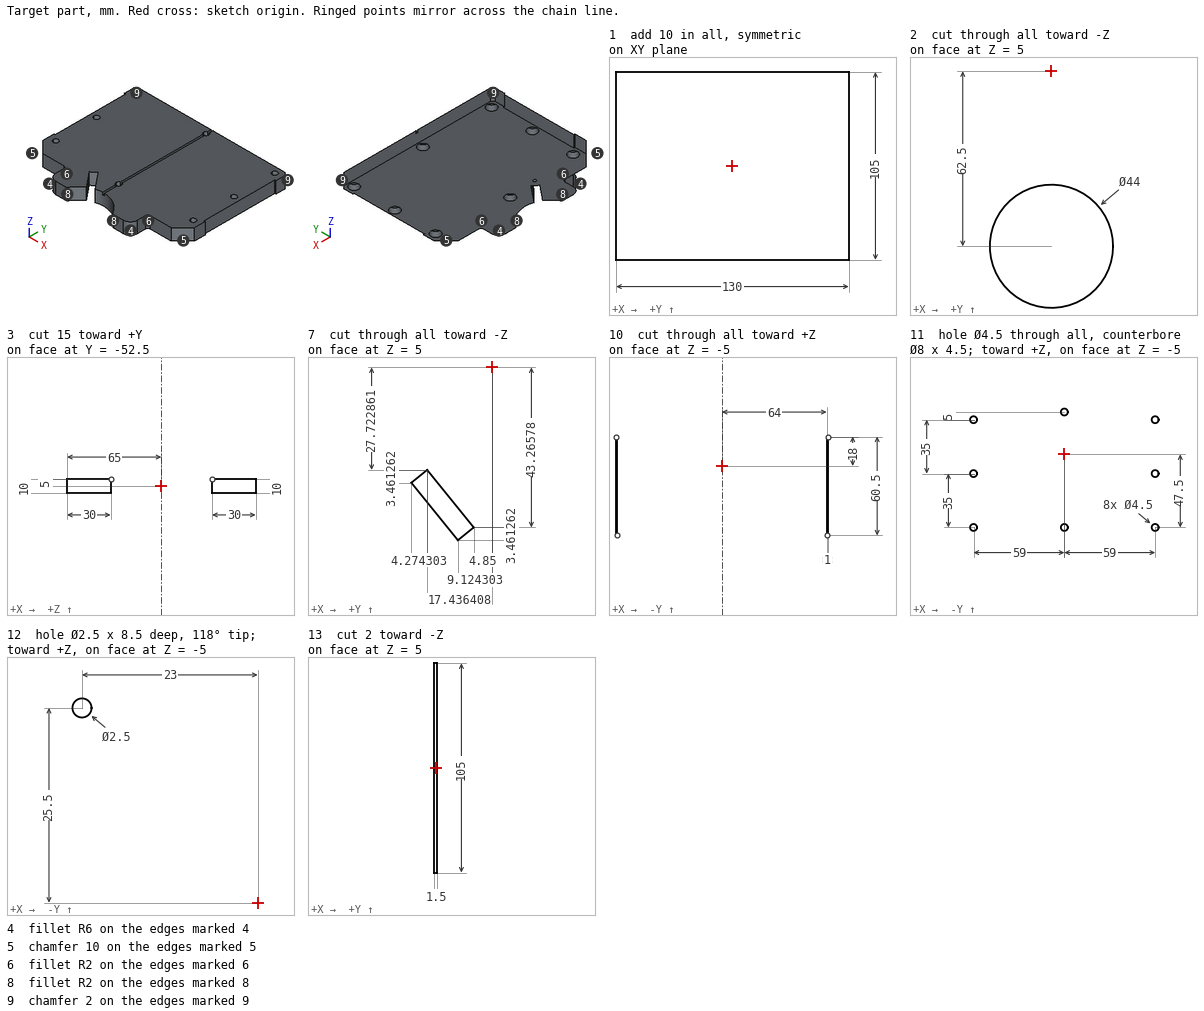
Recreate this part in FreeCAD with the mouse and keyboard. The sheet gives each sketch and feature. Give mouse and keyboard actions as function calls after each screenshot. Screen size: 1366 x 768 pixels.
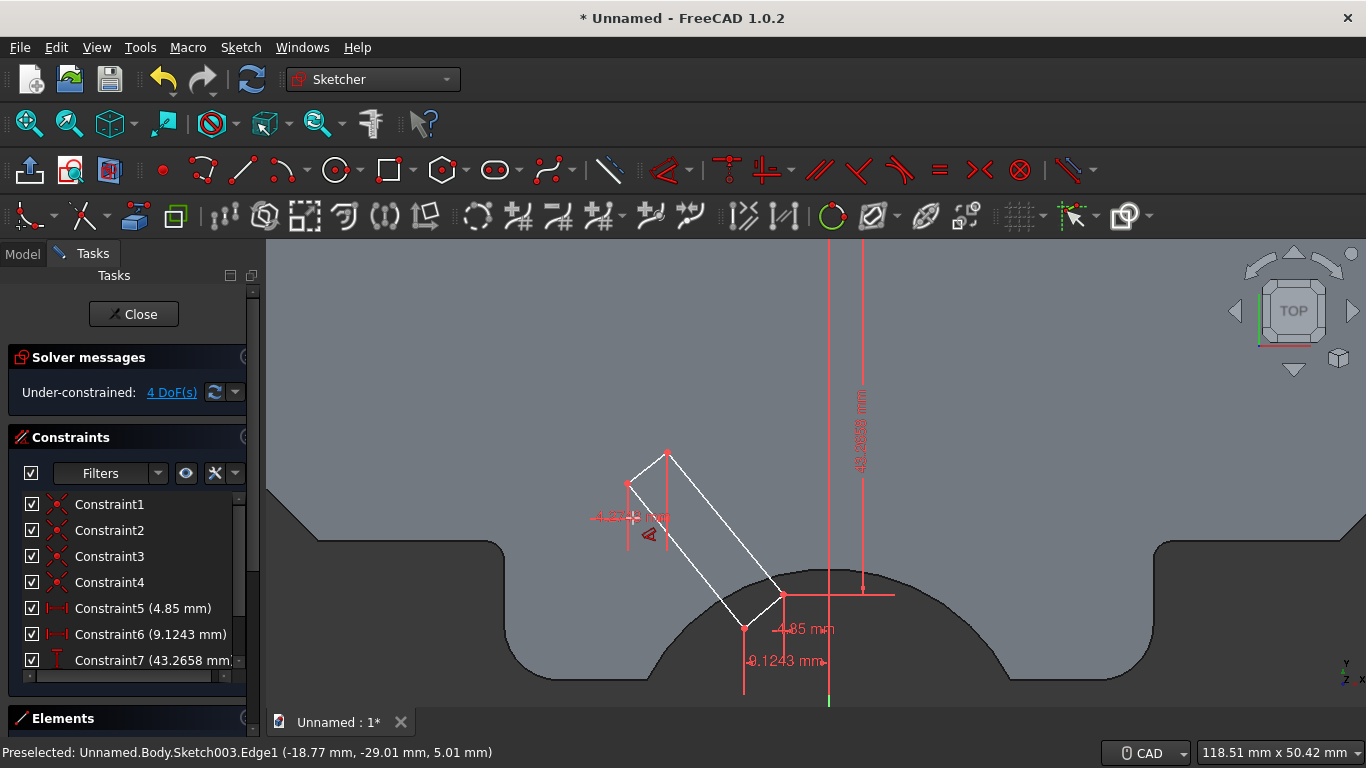
scroll(656, 462, up, 2)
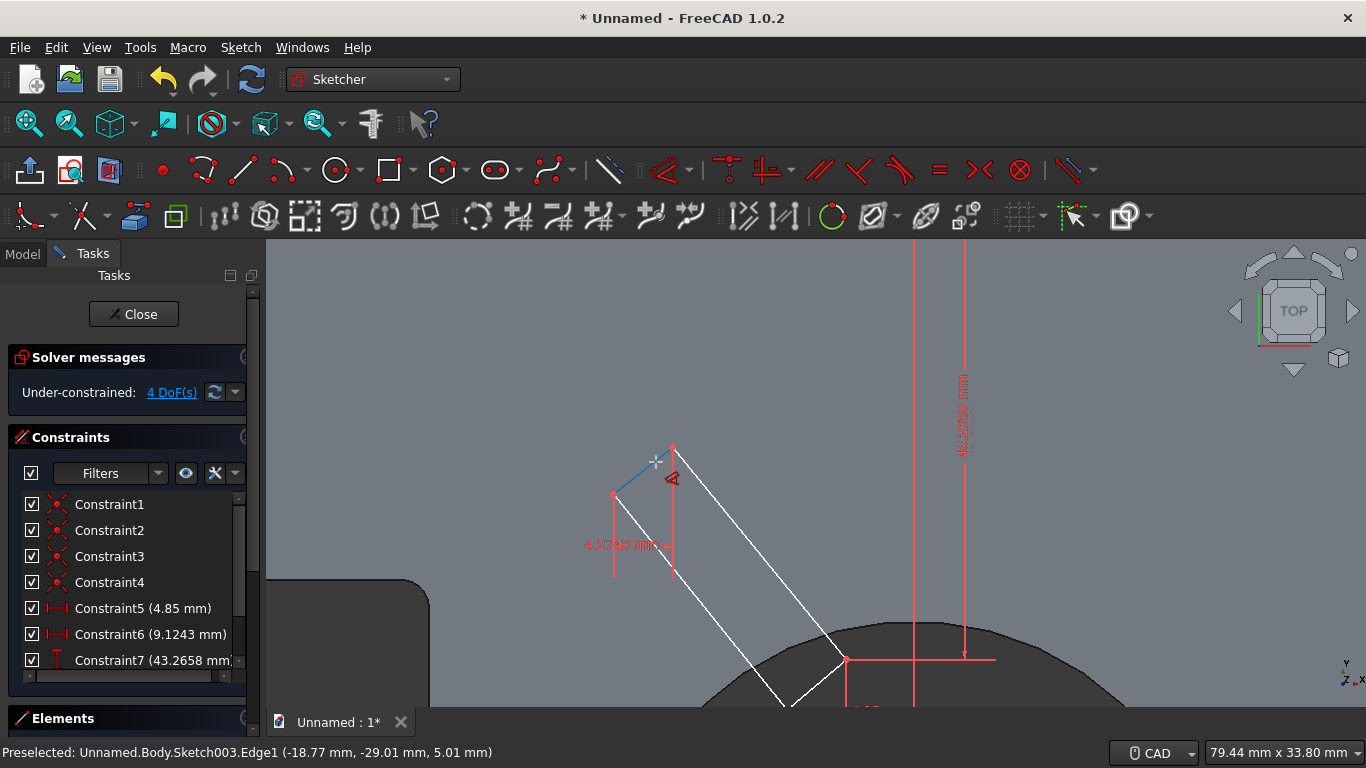
click(655, 461)
click(580, 471)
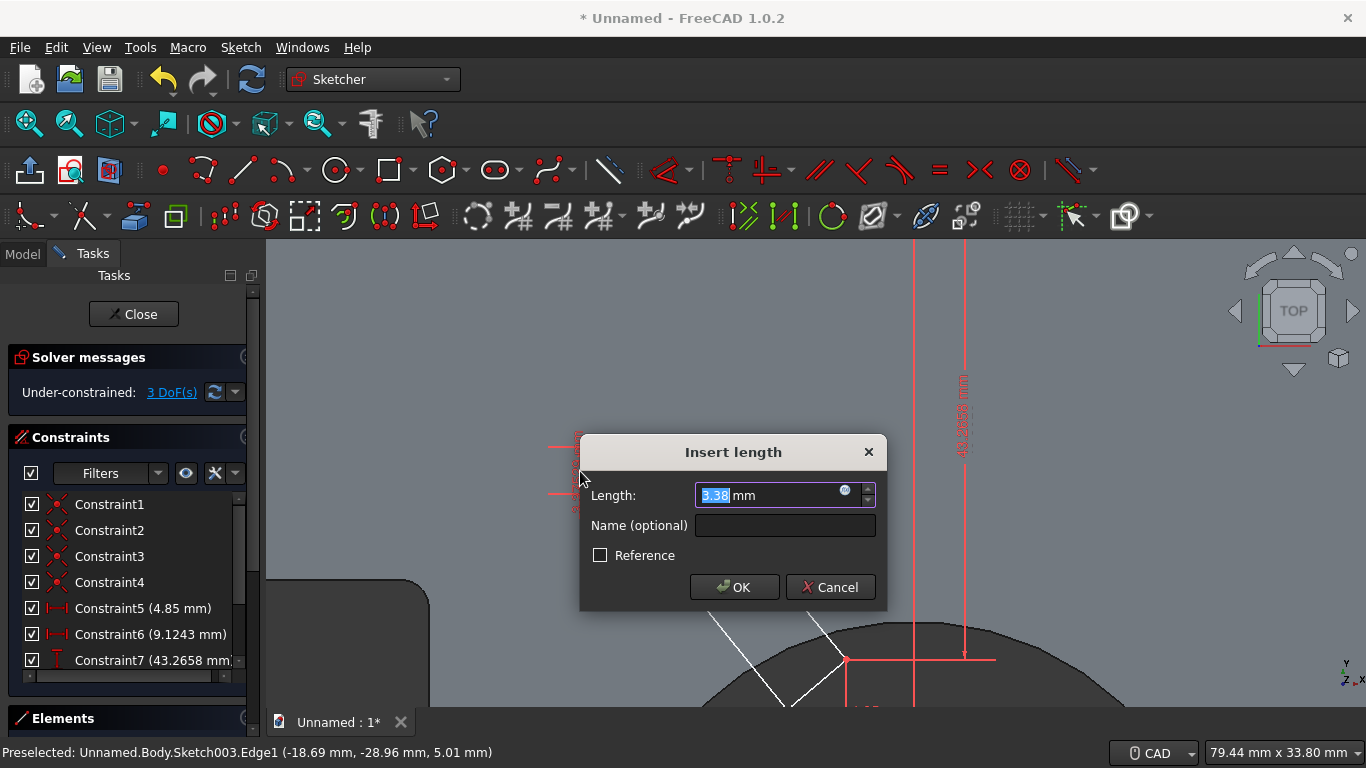
text(3.461262)
key(Return)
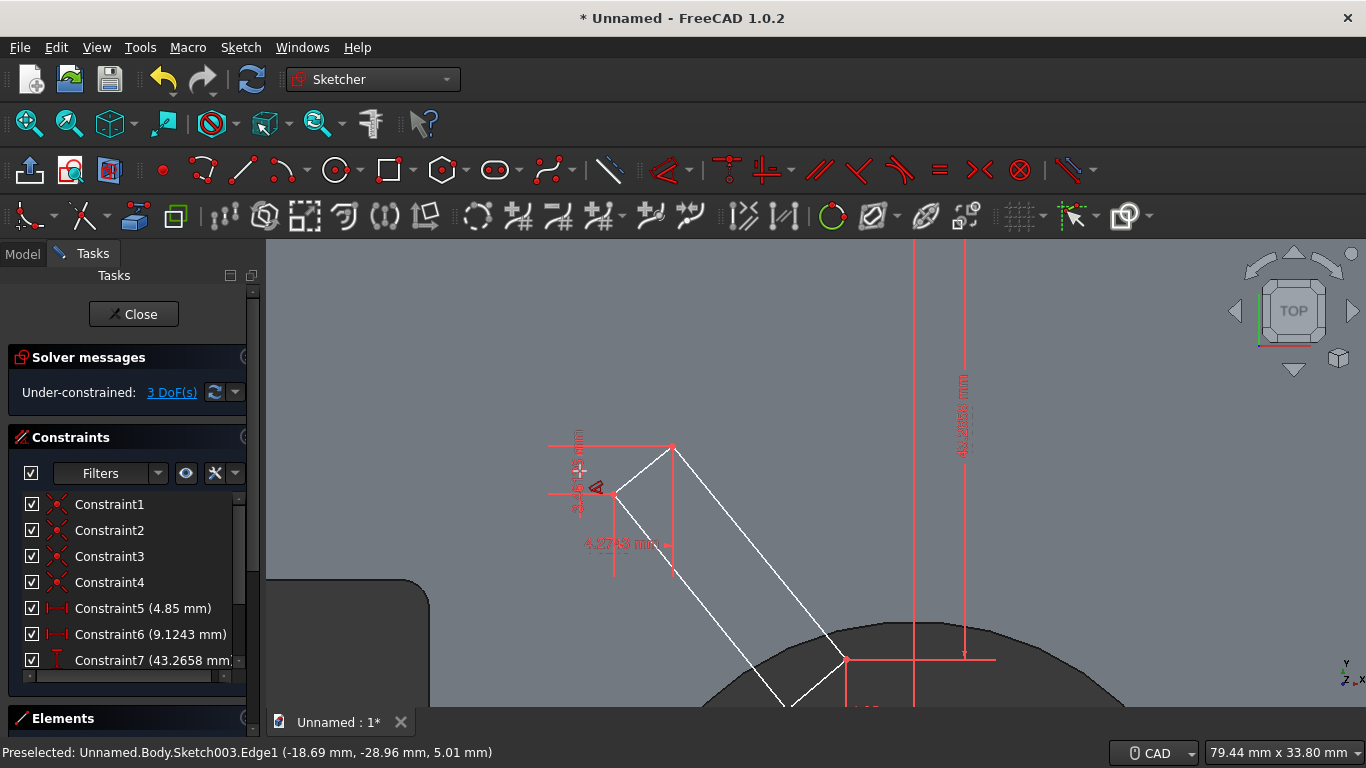
click(829, 675)
click(880, 669)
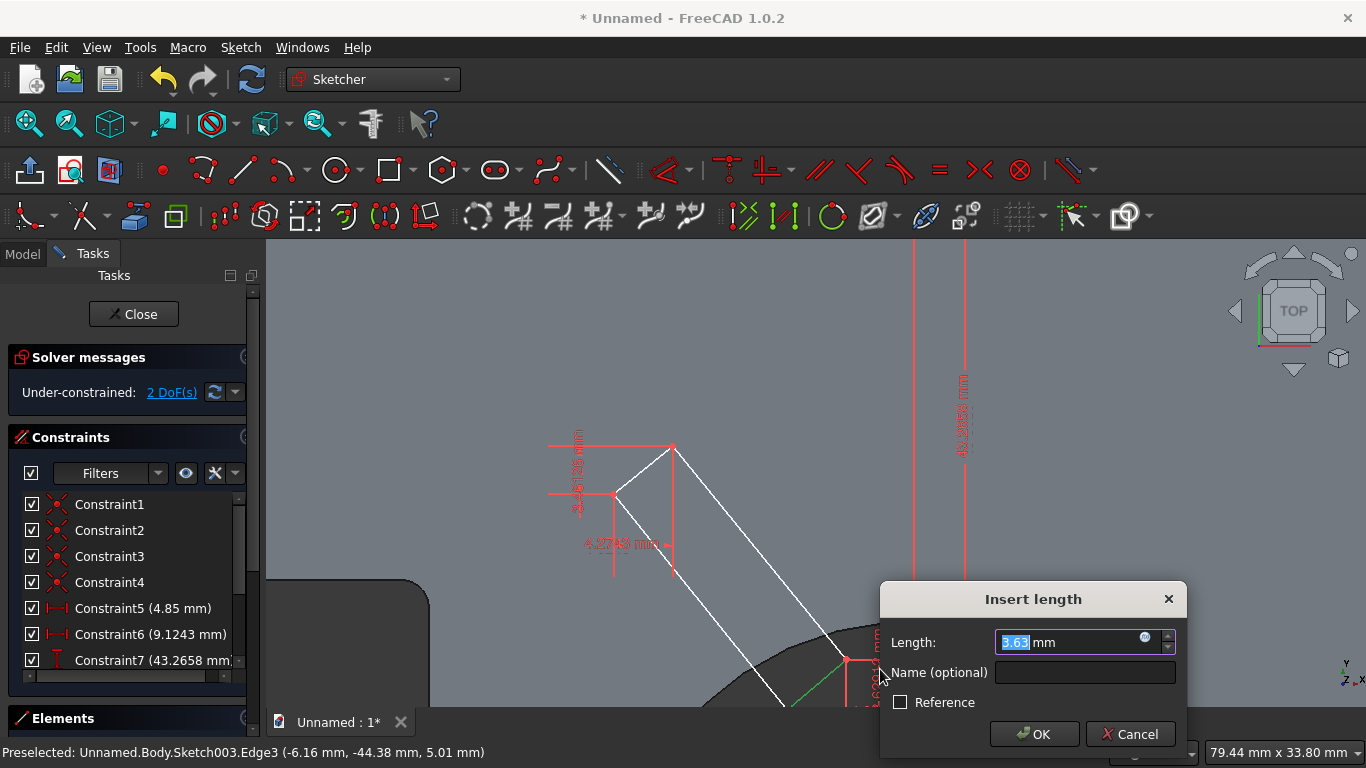
text(3.461262)
key(Return)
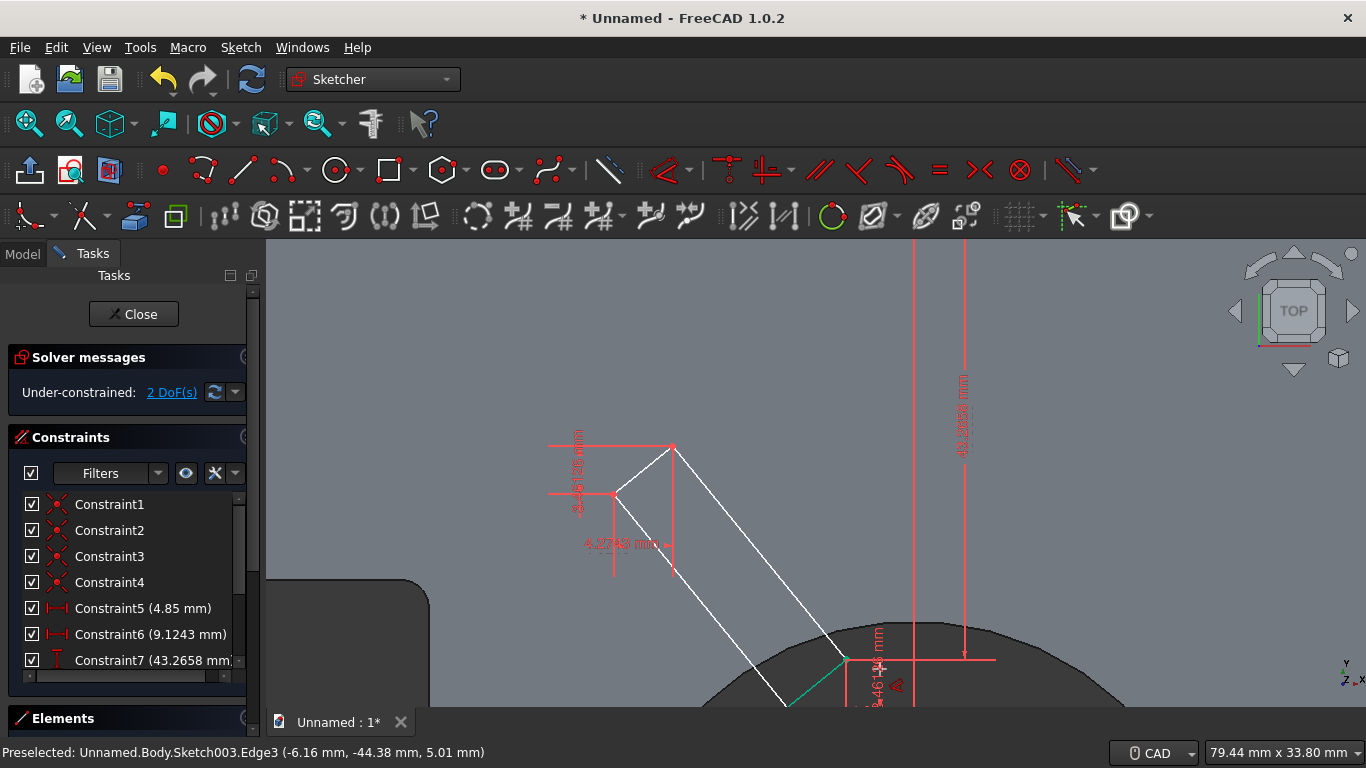
click(673, 446)
click(793, 480)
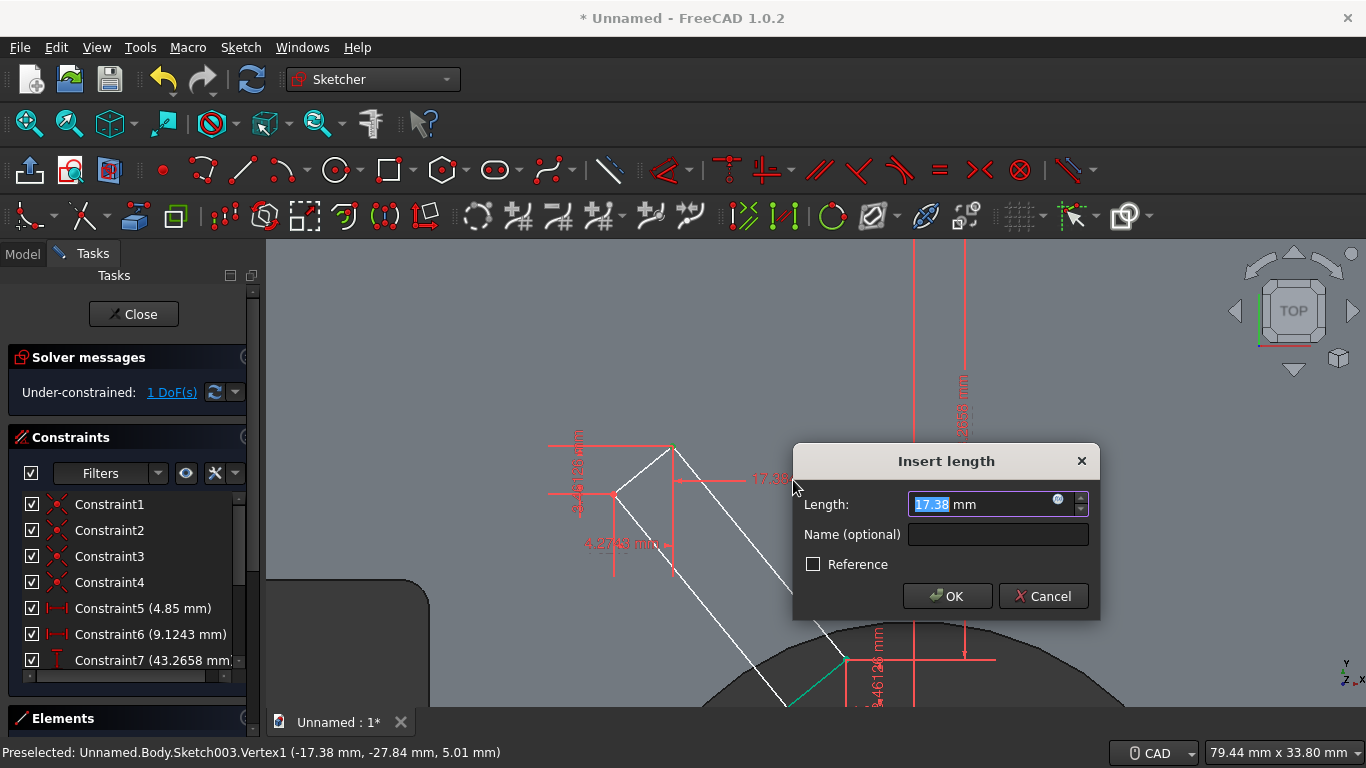
text(17.436408)
key(Return)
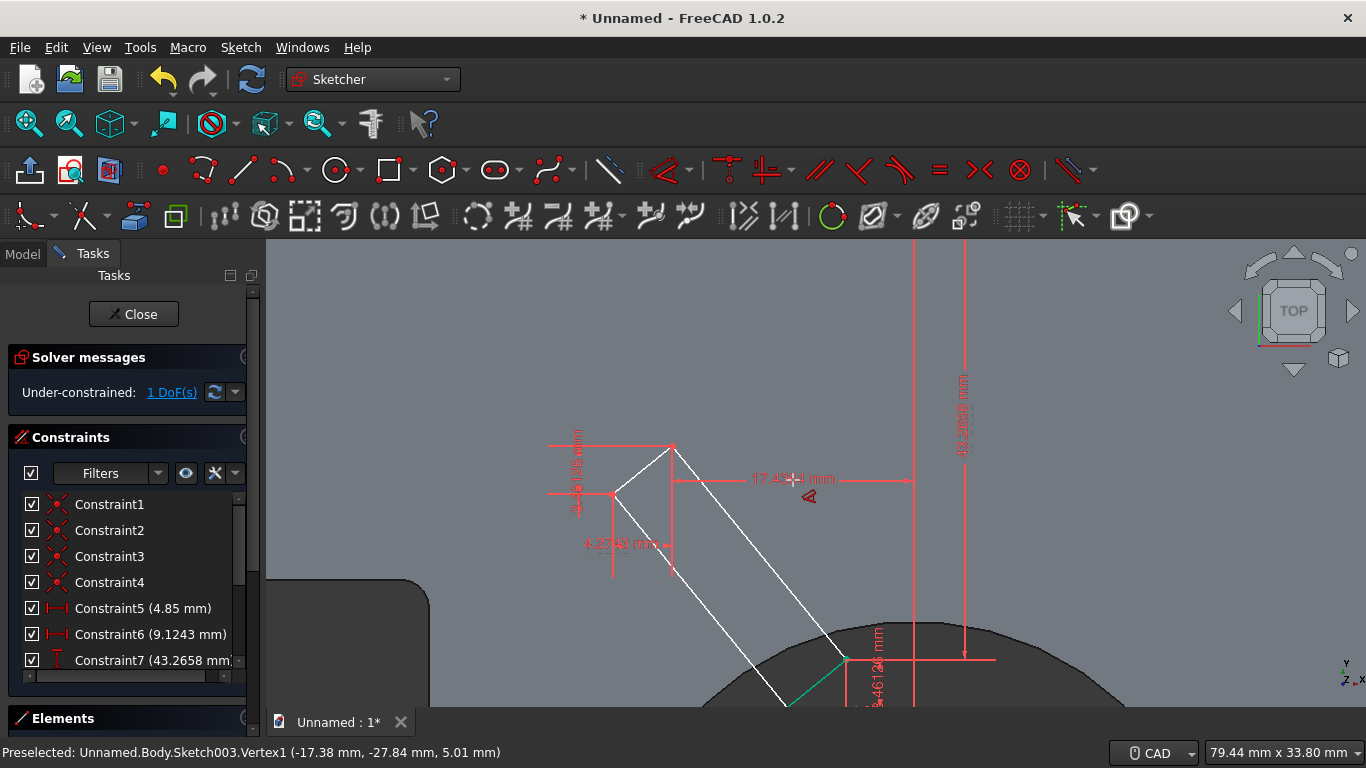
click(672, 446)
click(948, 357)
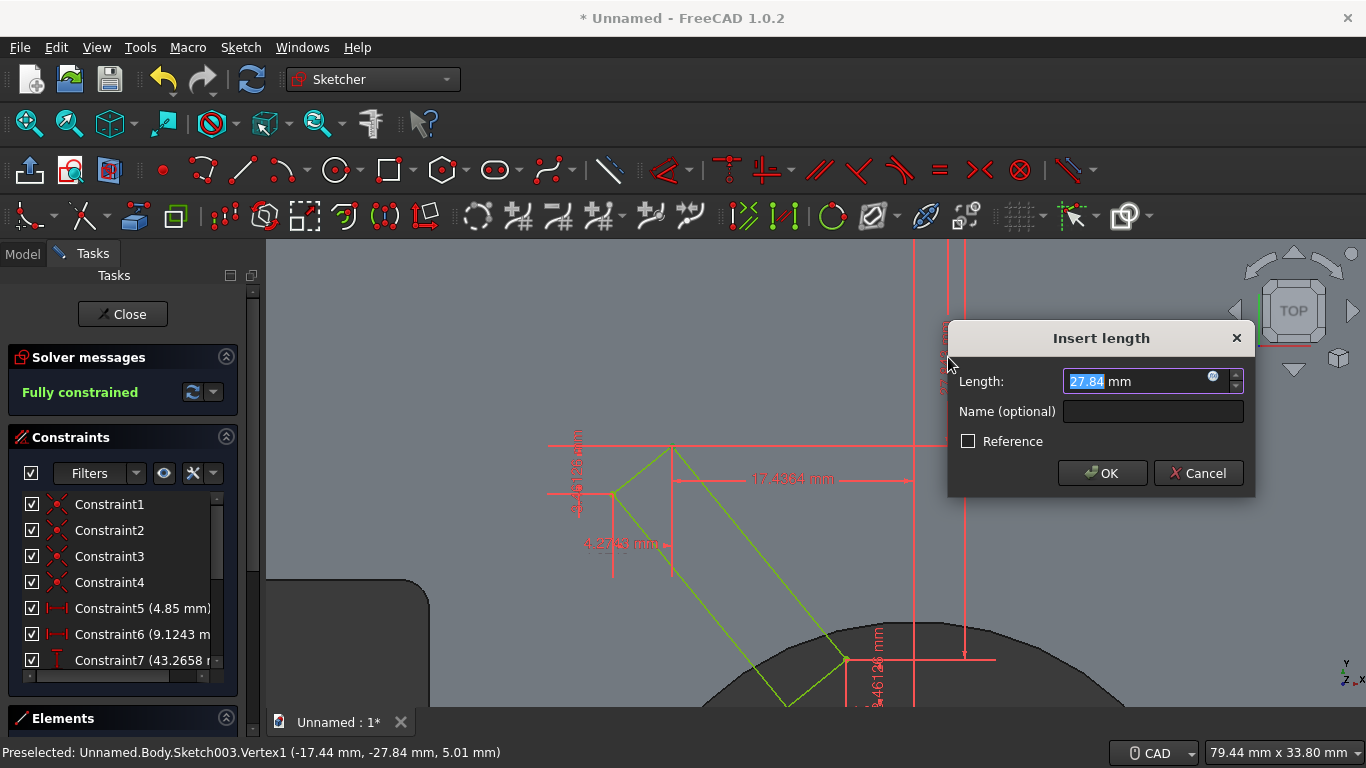
text(27.722861)
key(Return)
key(Escape)